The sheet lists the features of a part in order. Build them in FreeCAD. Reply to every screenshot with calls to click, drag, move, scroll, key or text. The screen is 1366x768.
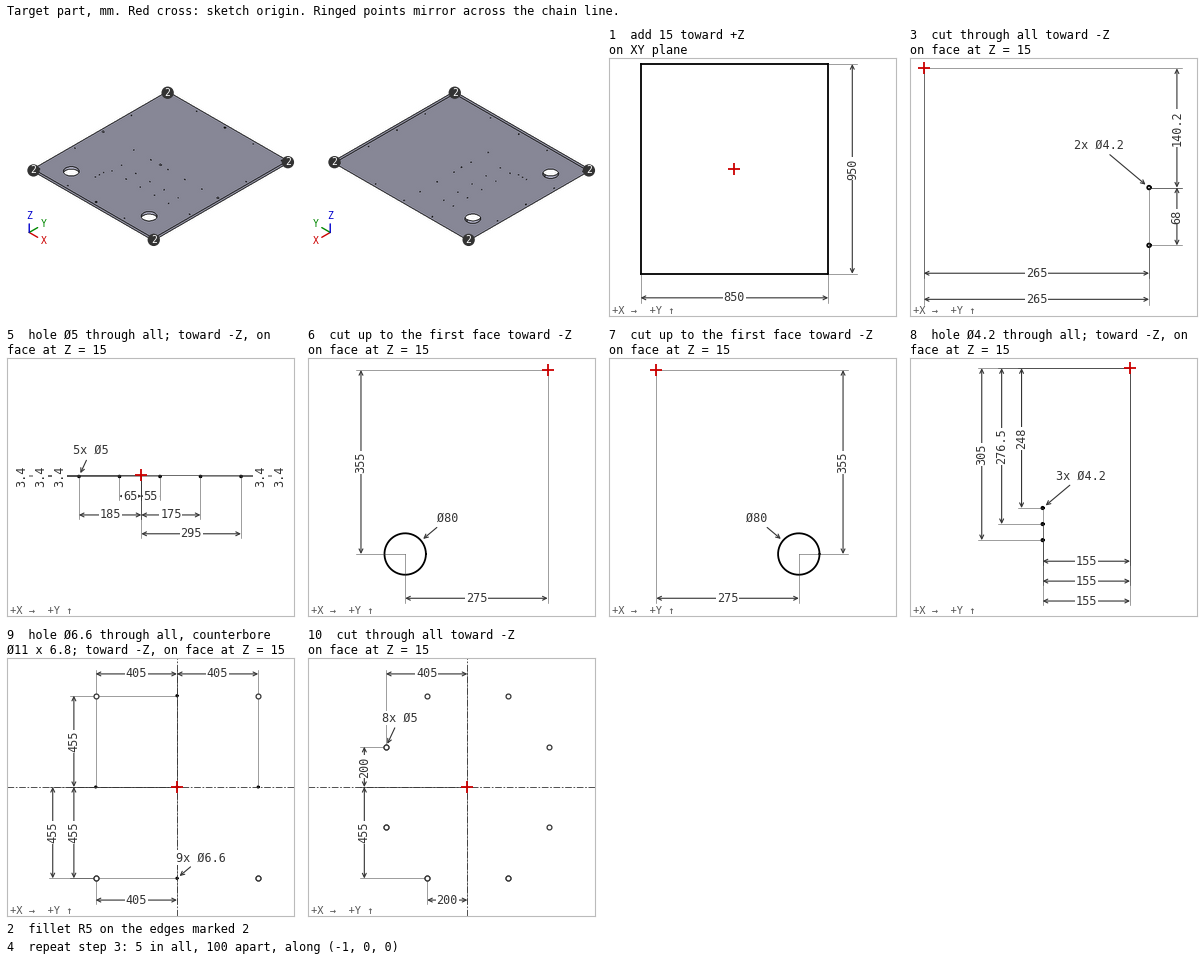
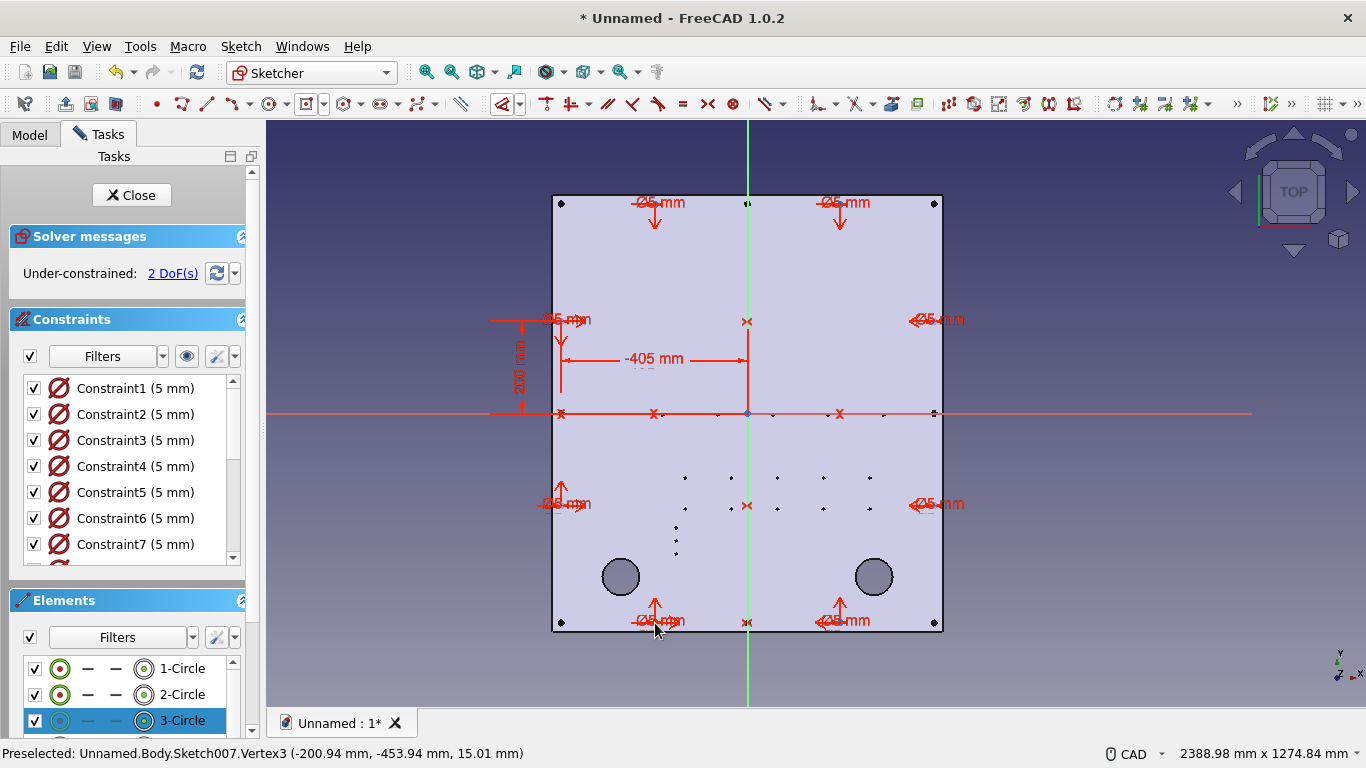
key(l)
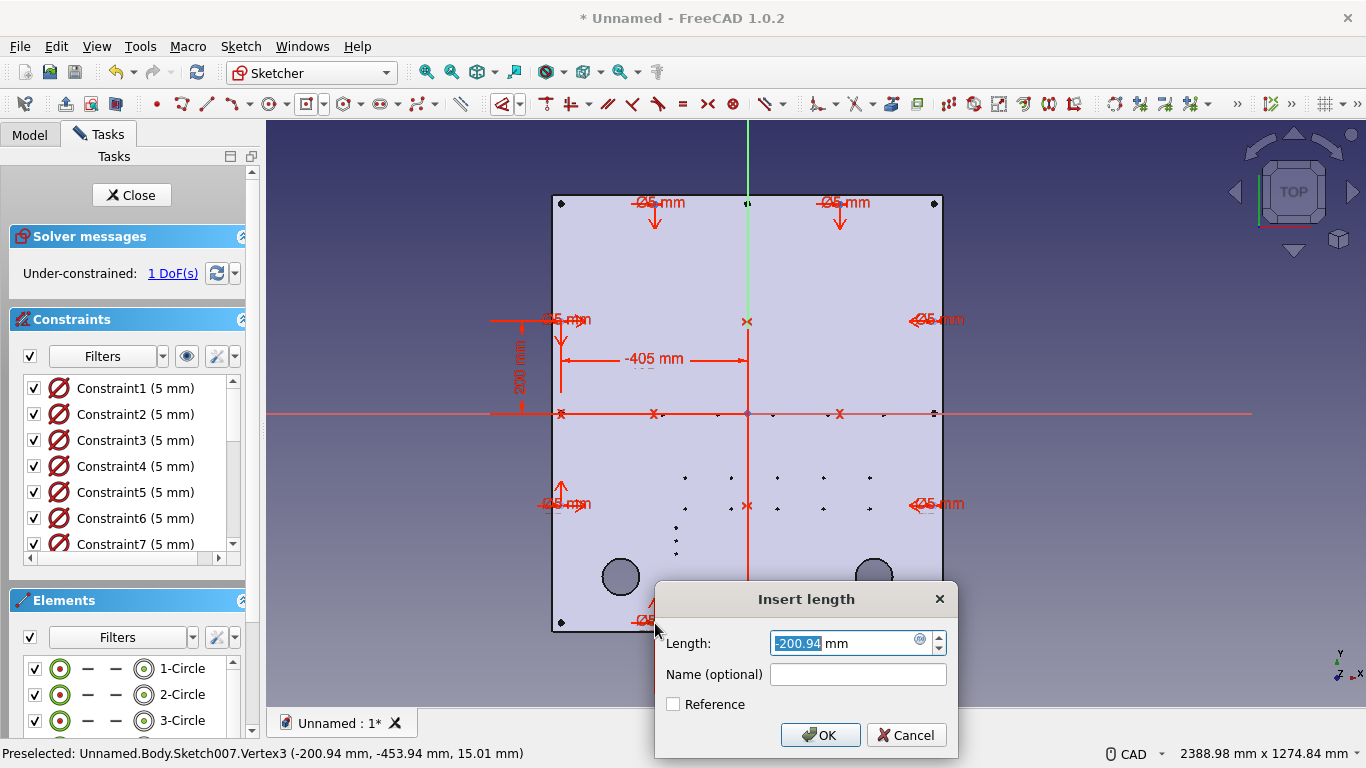
text(-200)
key(Return)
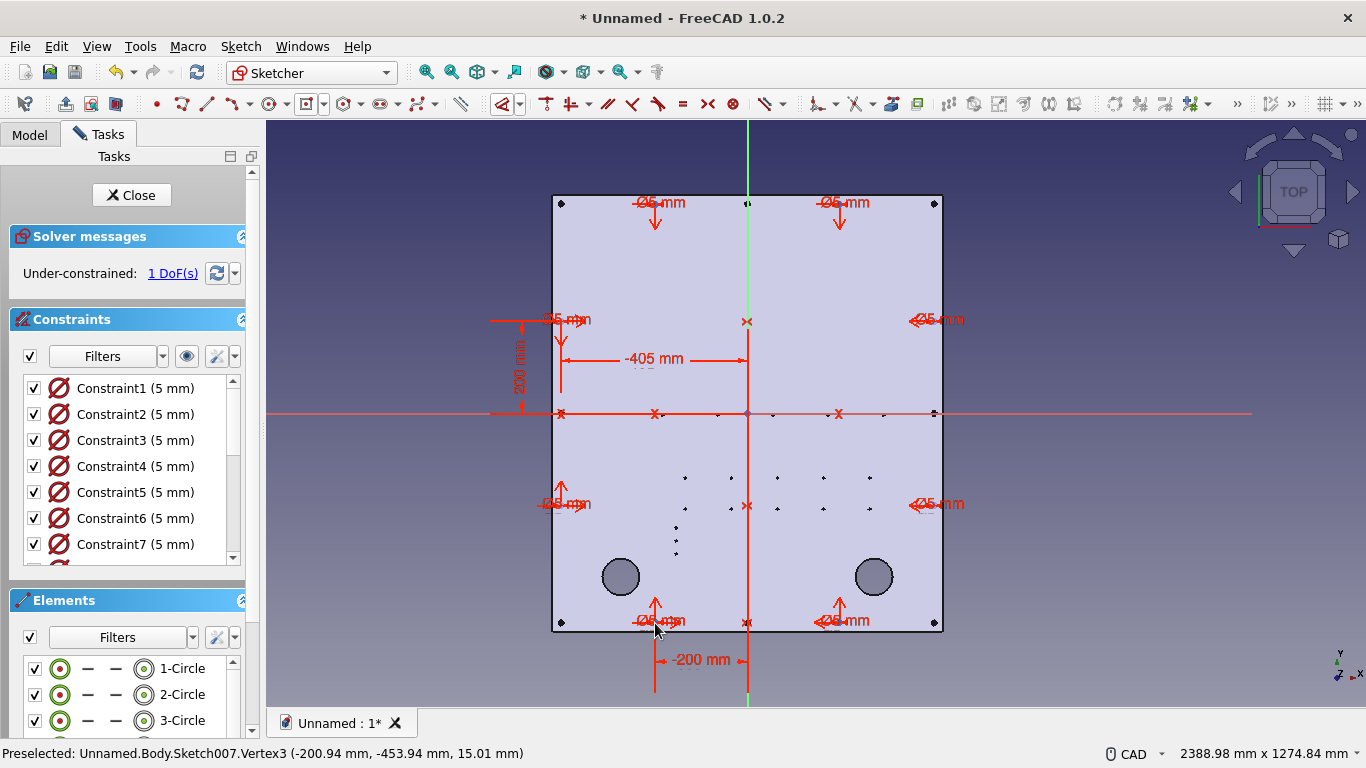
click(655, 623)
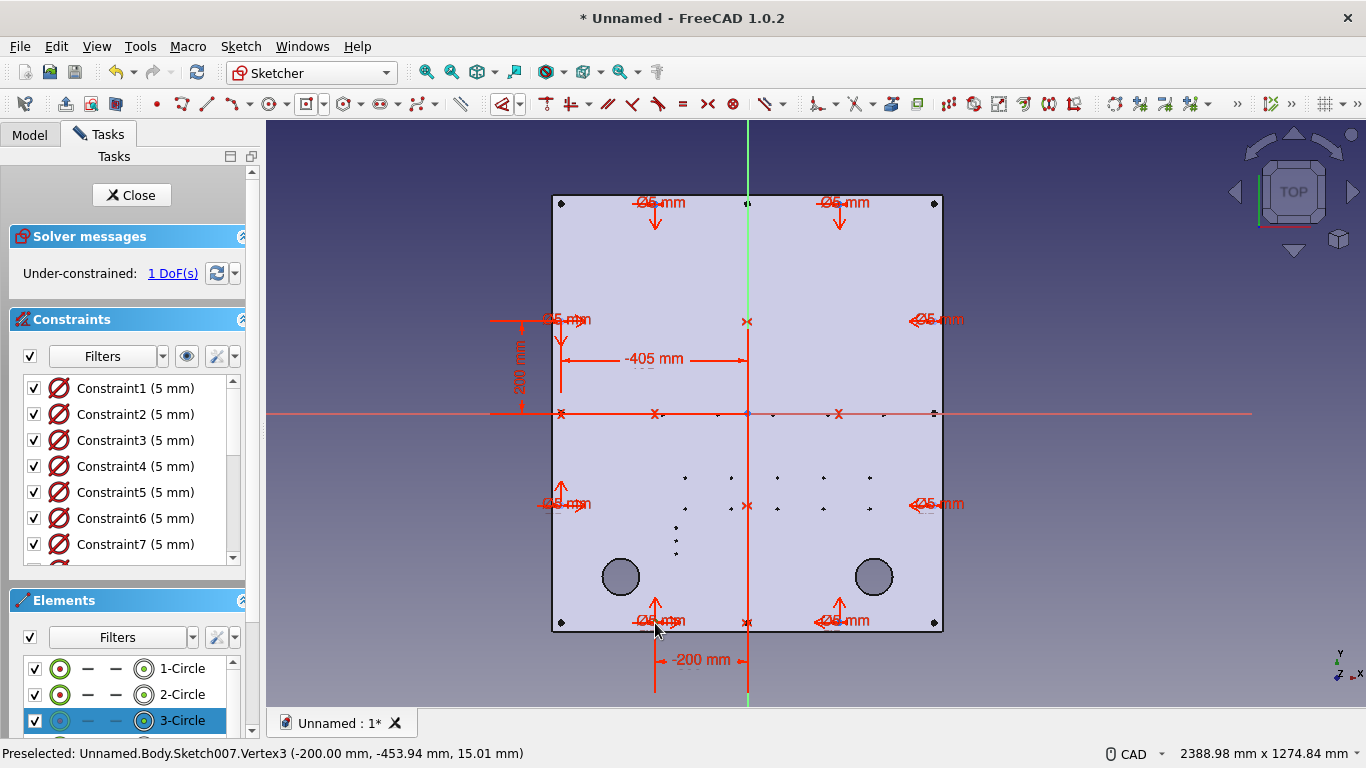
click(520, 104)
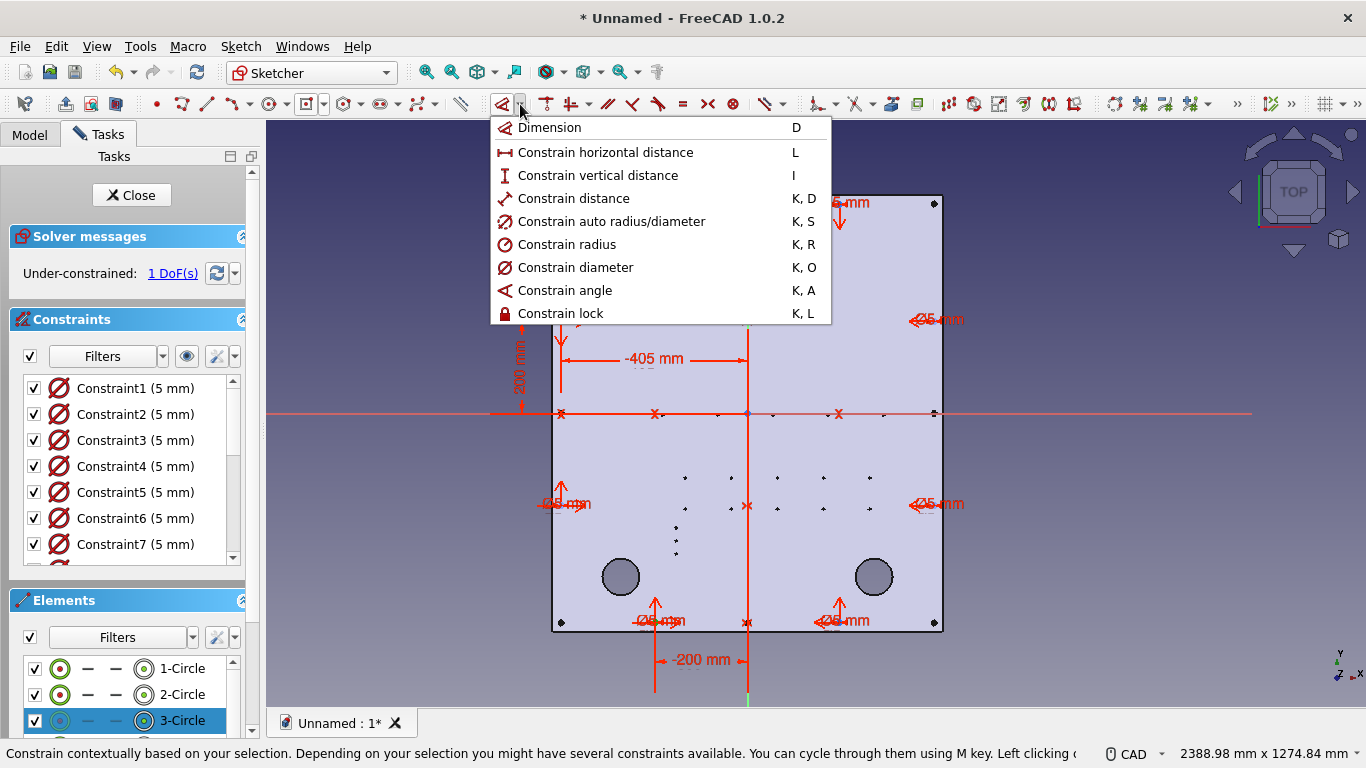
click(661, 176)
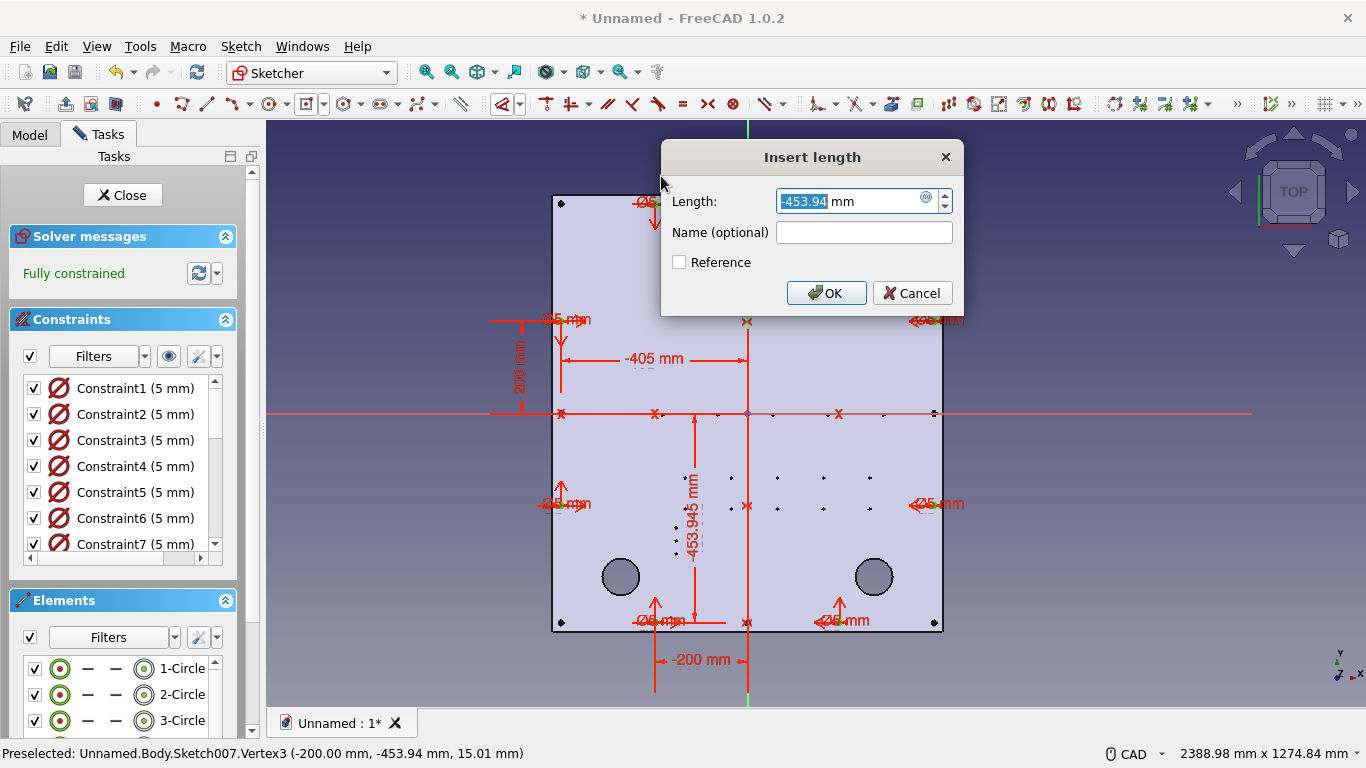
text(-455)
key(Return)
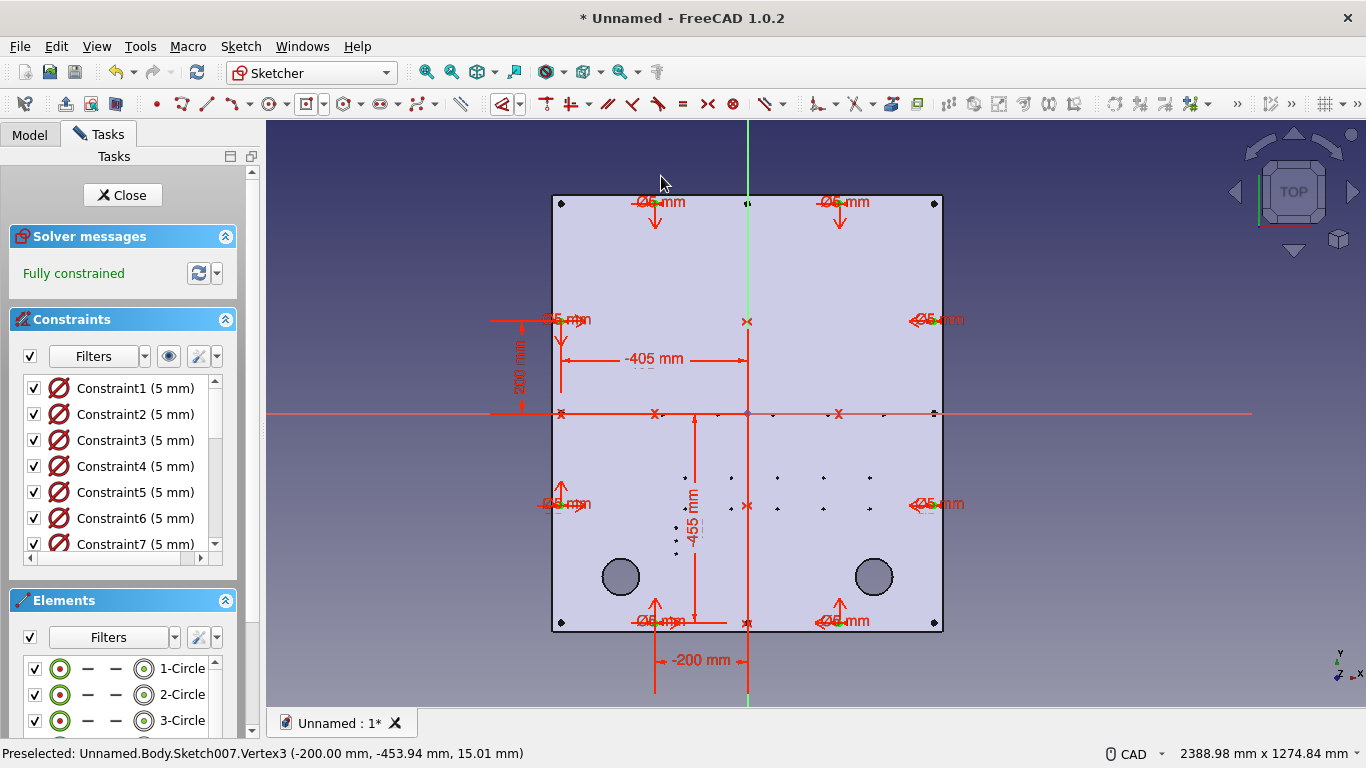
click(123, 195)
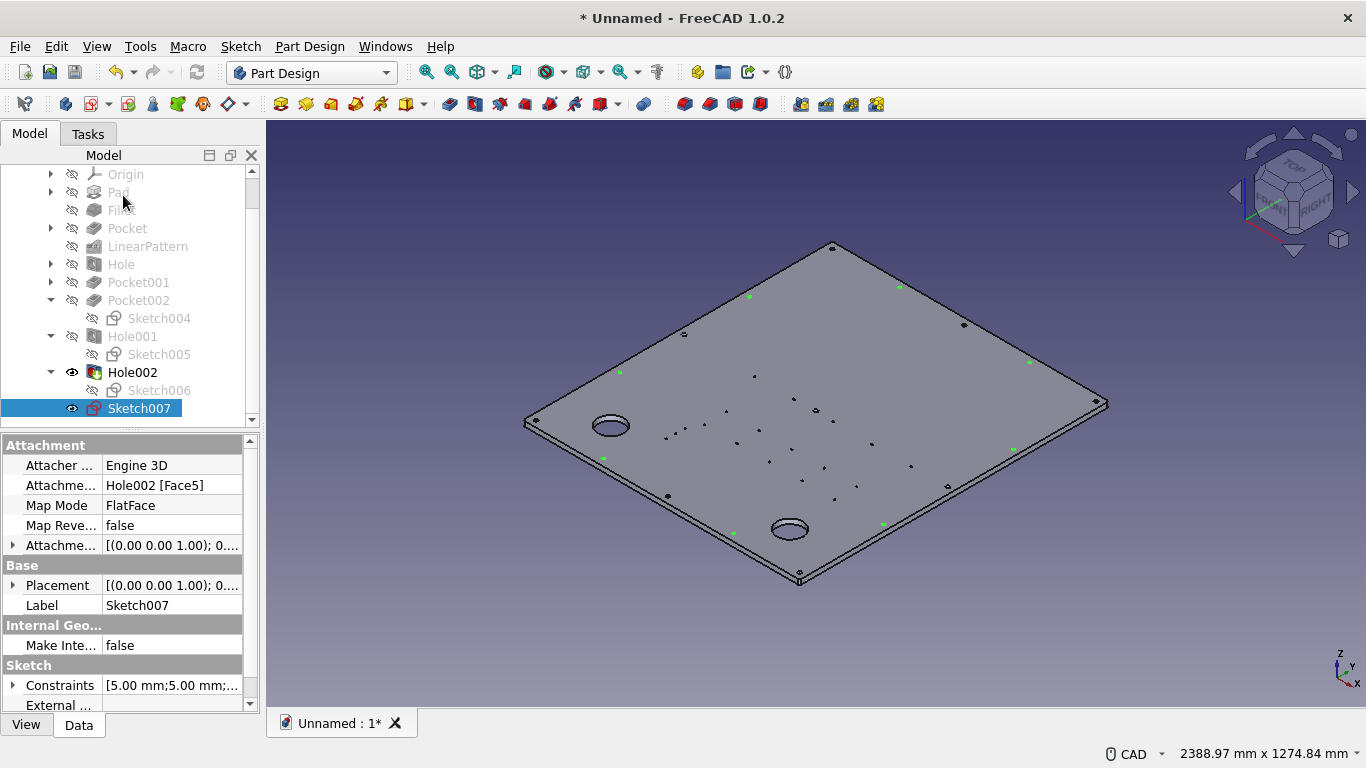
click(450, 104)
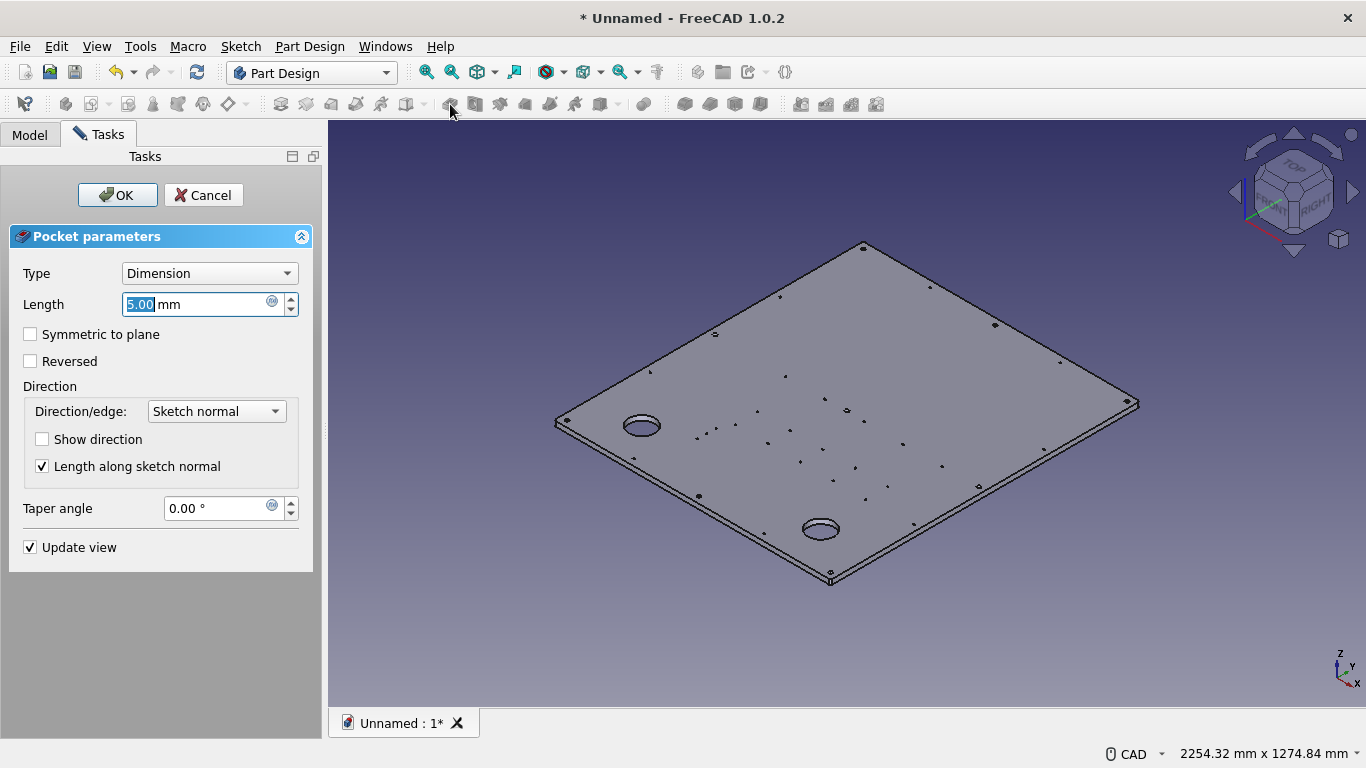
click(210, 274)